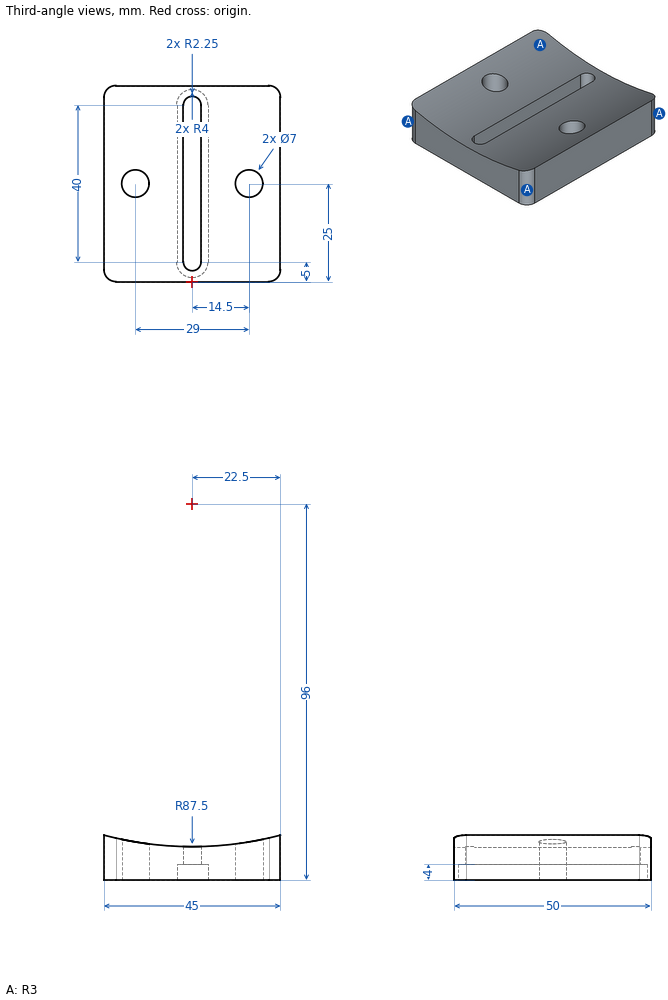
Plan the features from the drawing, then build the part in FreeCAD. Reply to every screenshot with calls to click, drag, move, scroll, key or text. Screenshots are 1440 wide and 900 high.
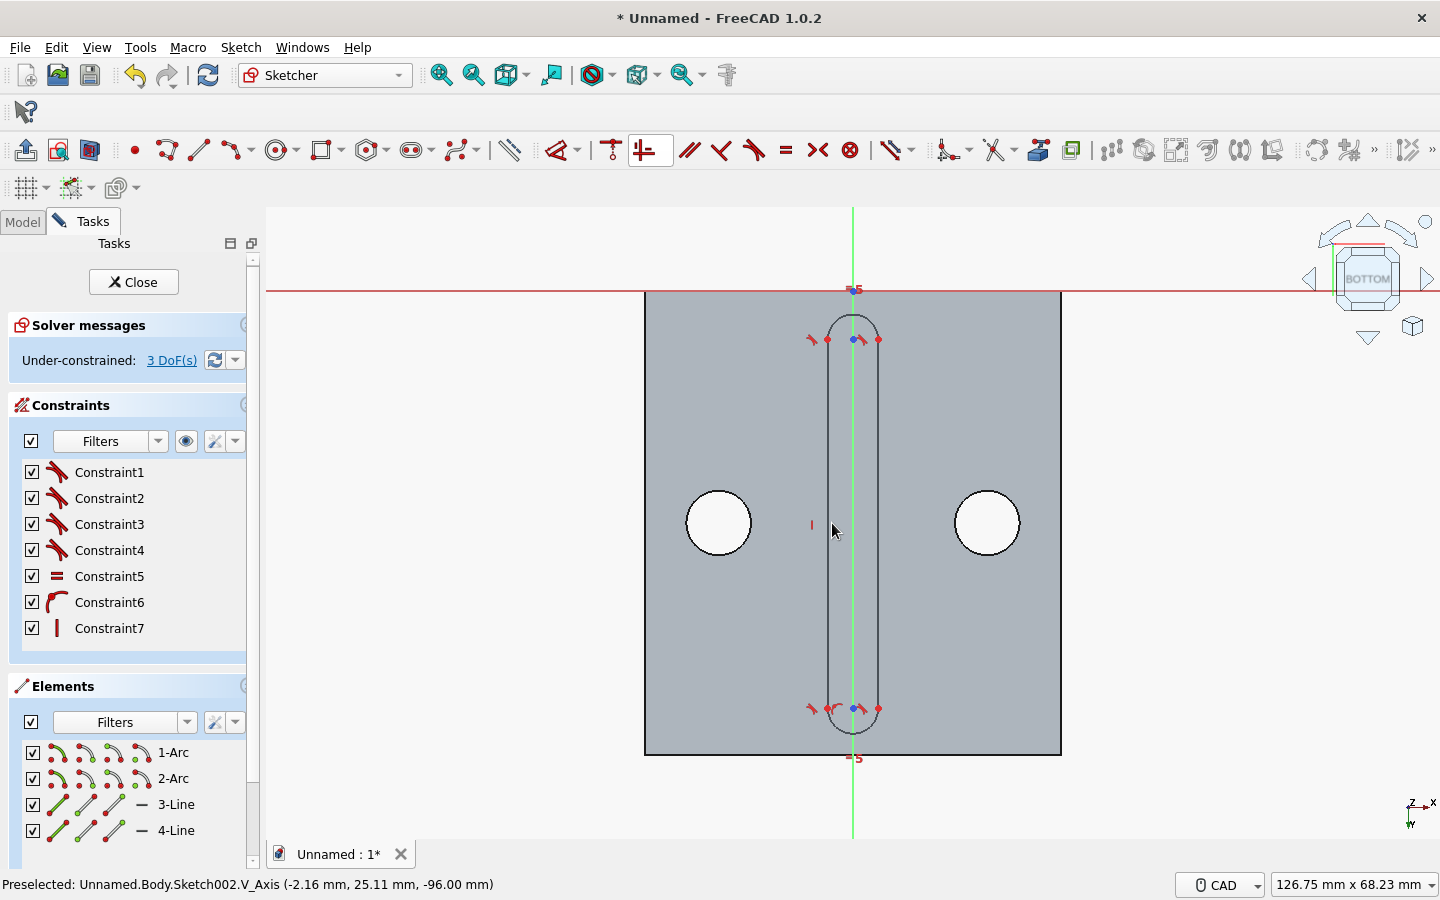
click(556, 150)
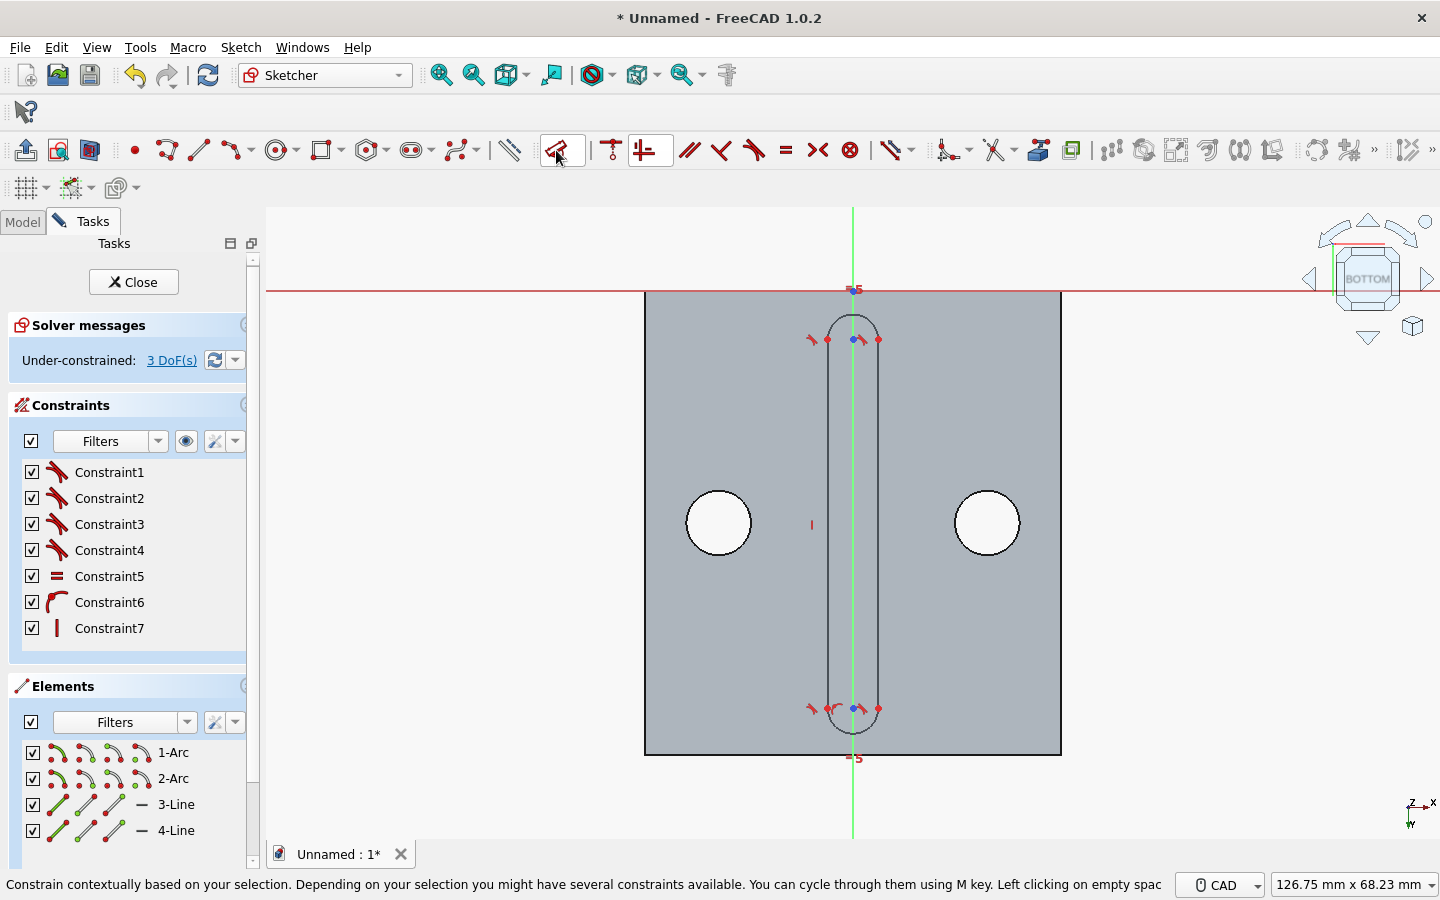
scroll(838, 729, up, 4)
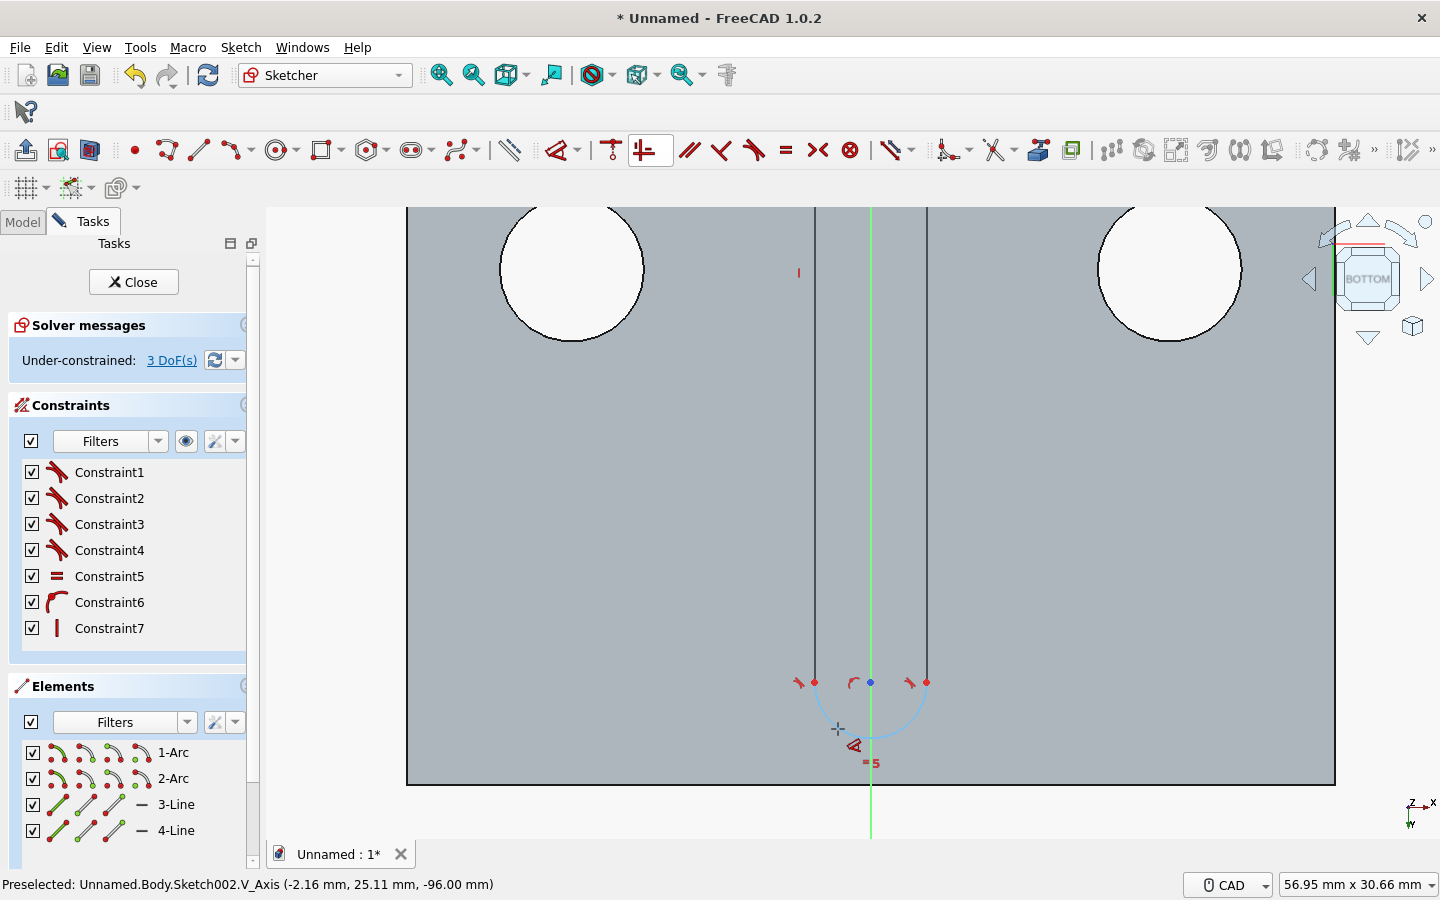
click(838, 728)
click(819, 754)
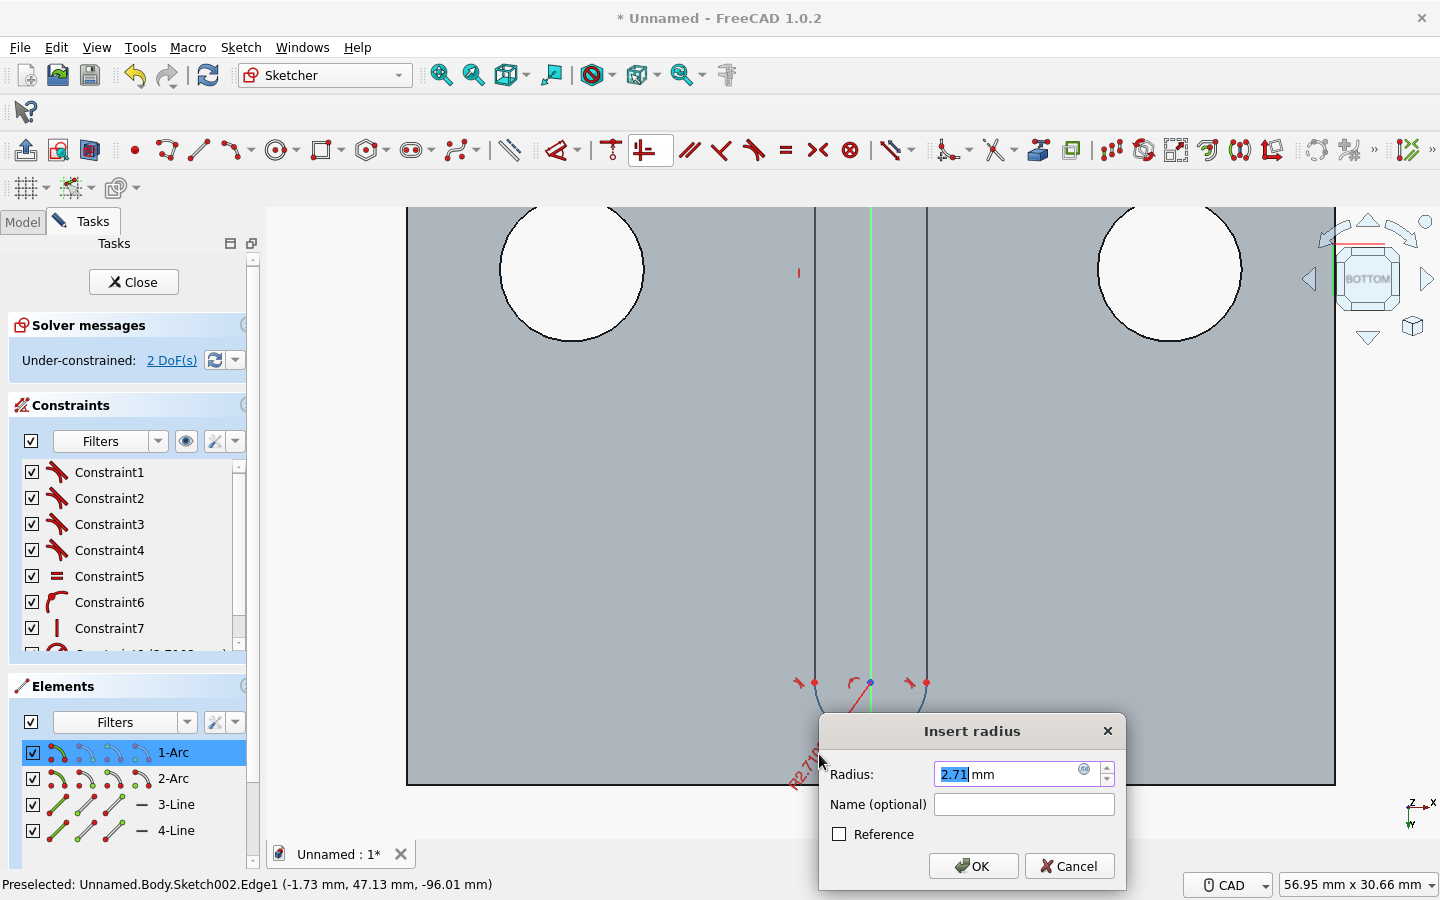
text(2.25)
key(Return)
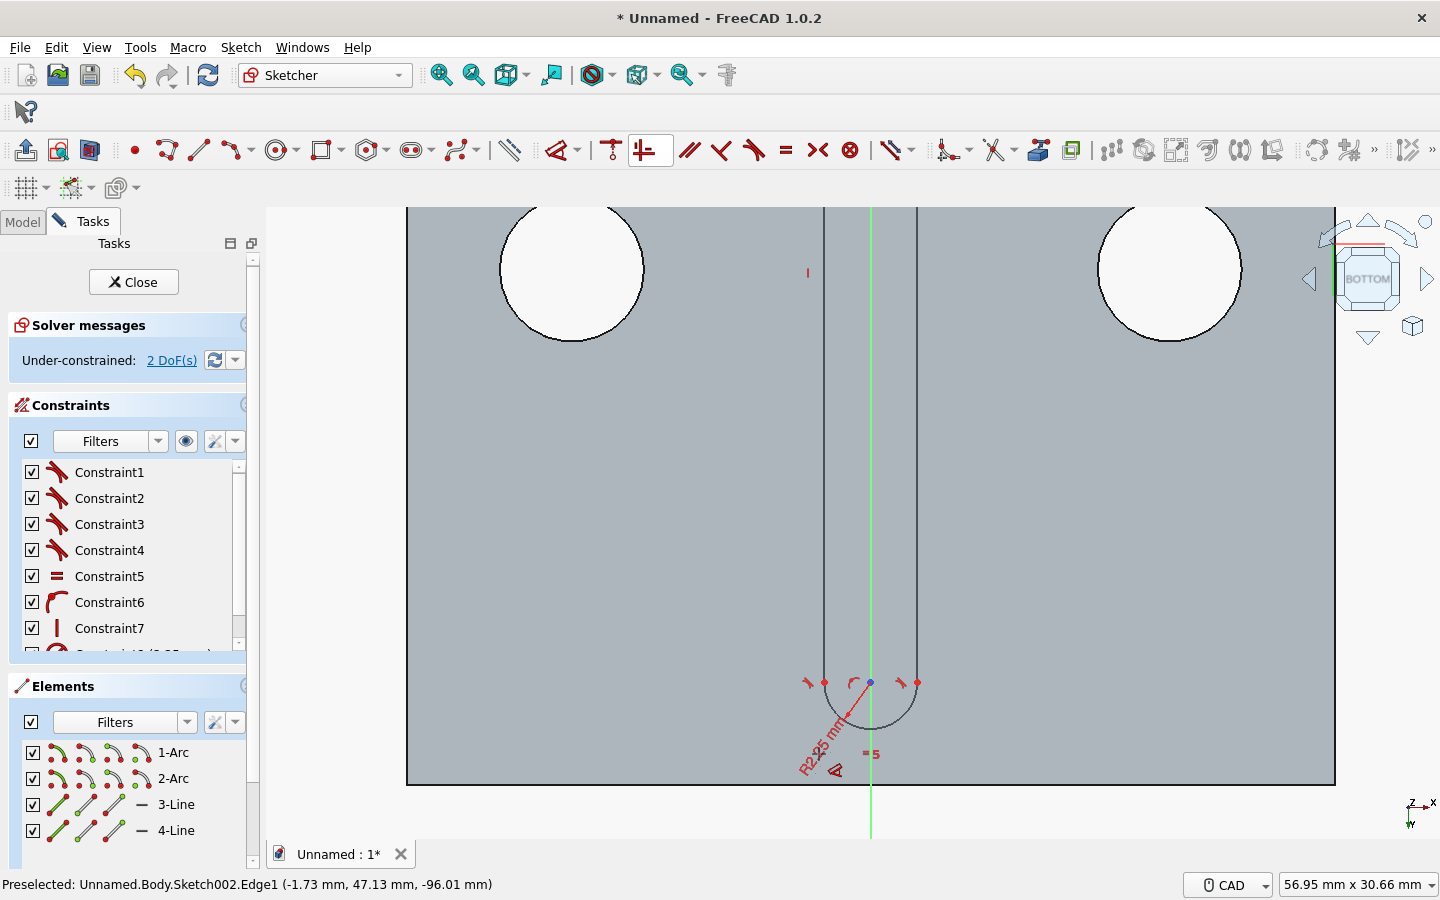
click(824, 436)
click(790, 459)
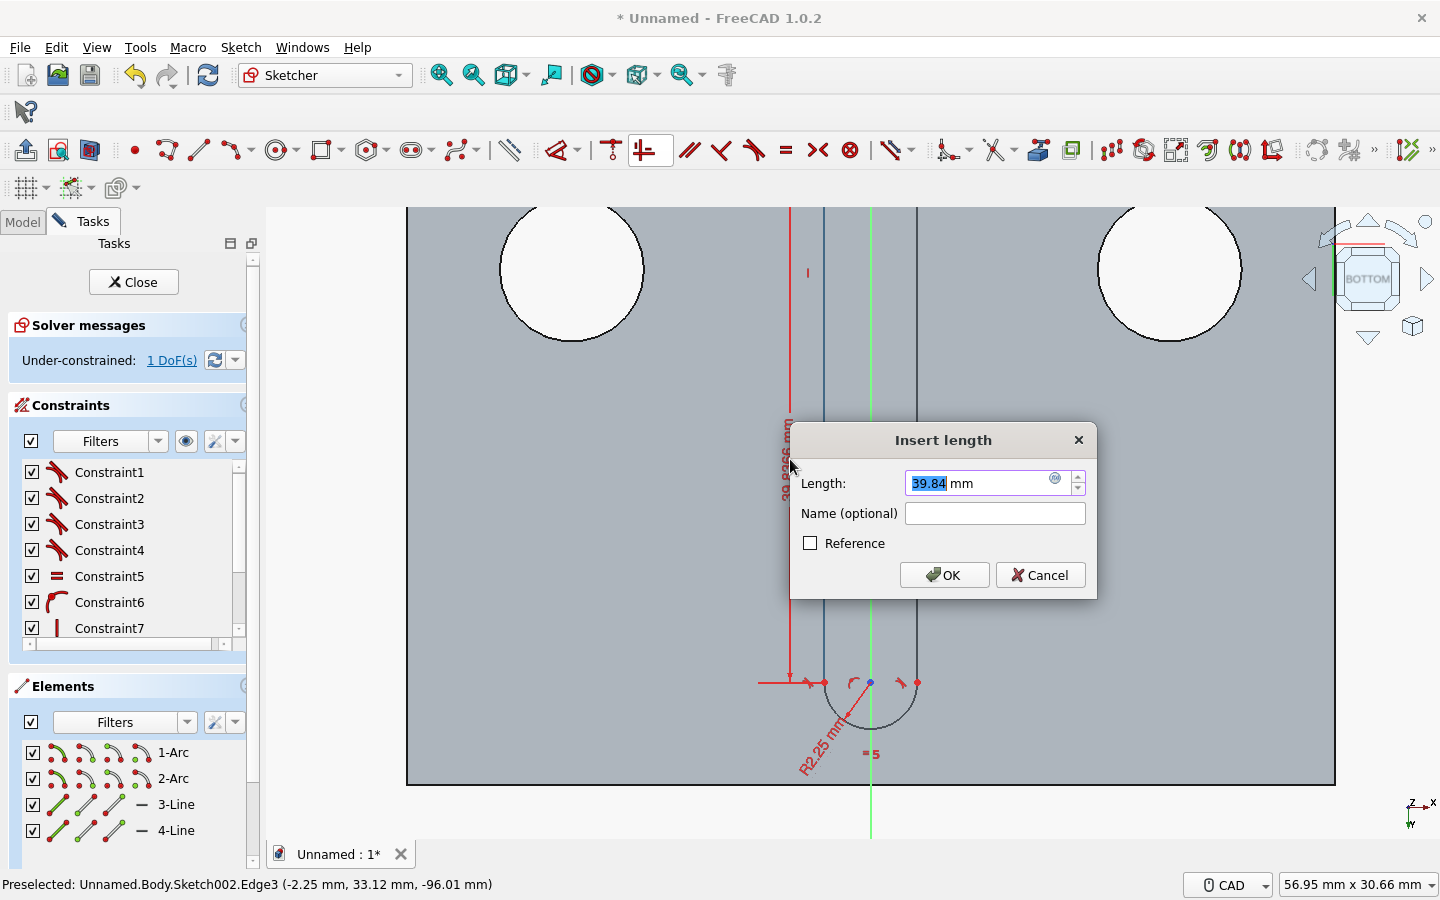
text(40)
key(Return)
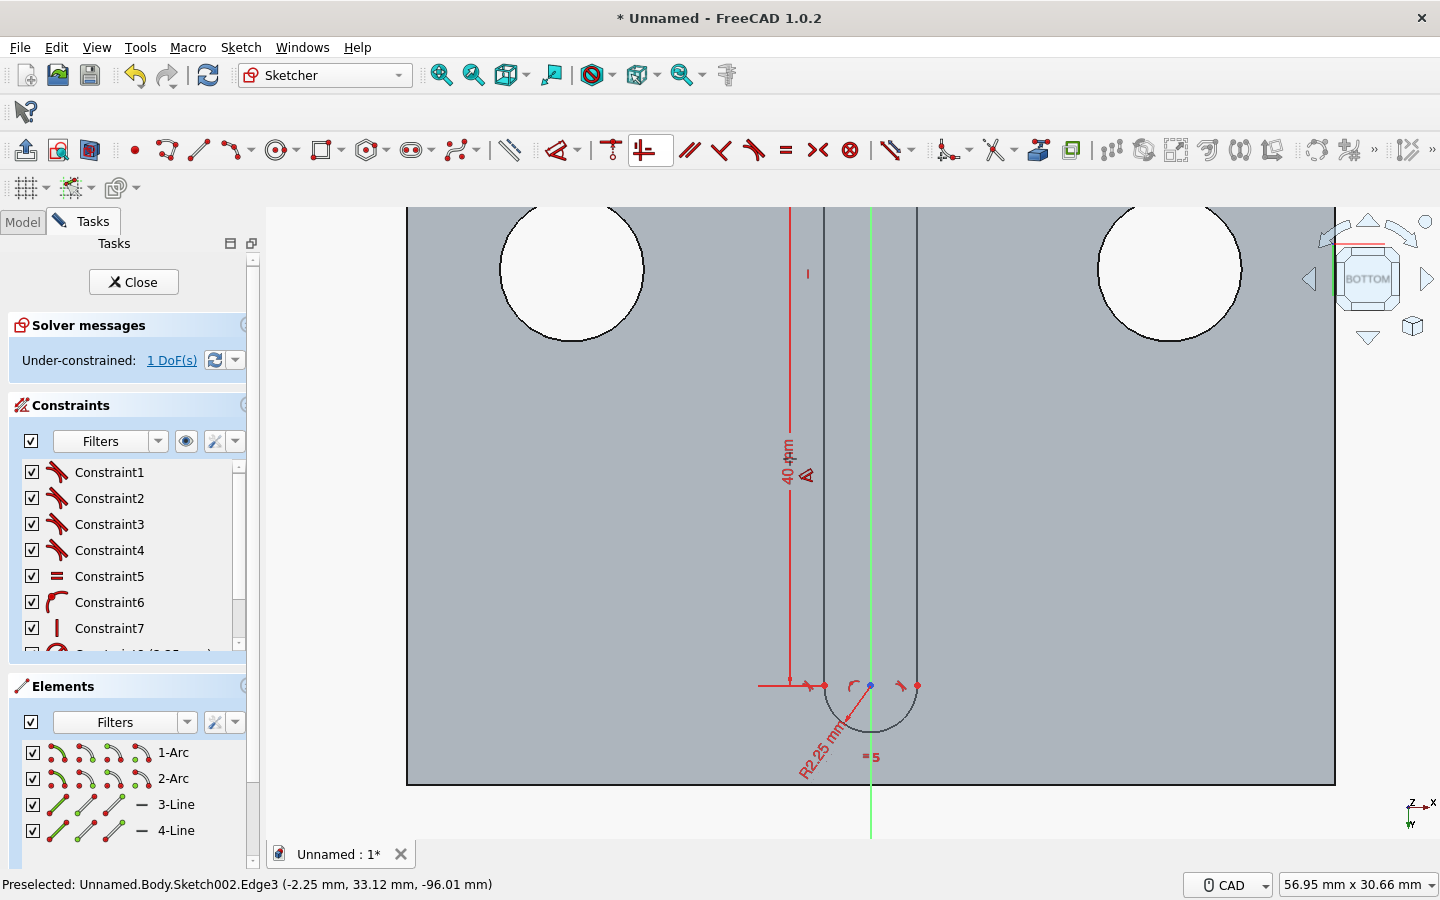
scroll(714, 753, down, 4)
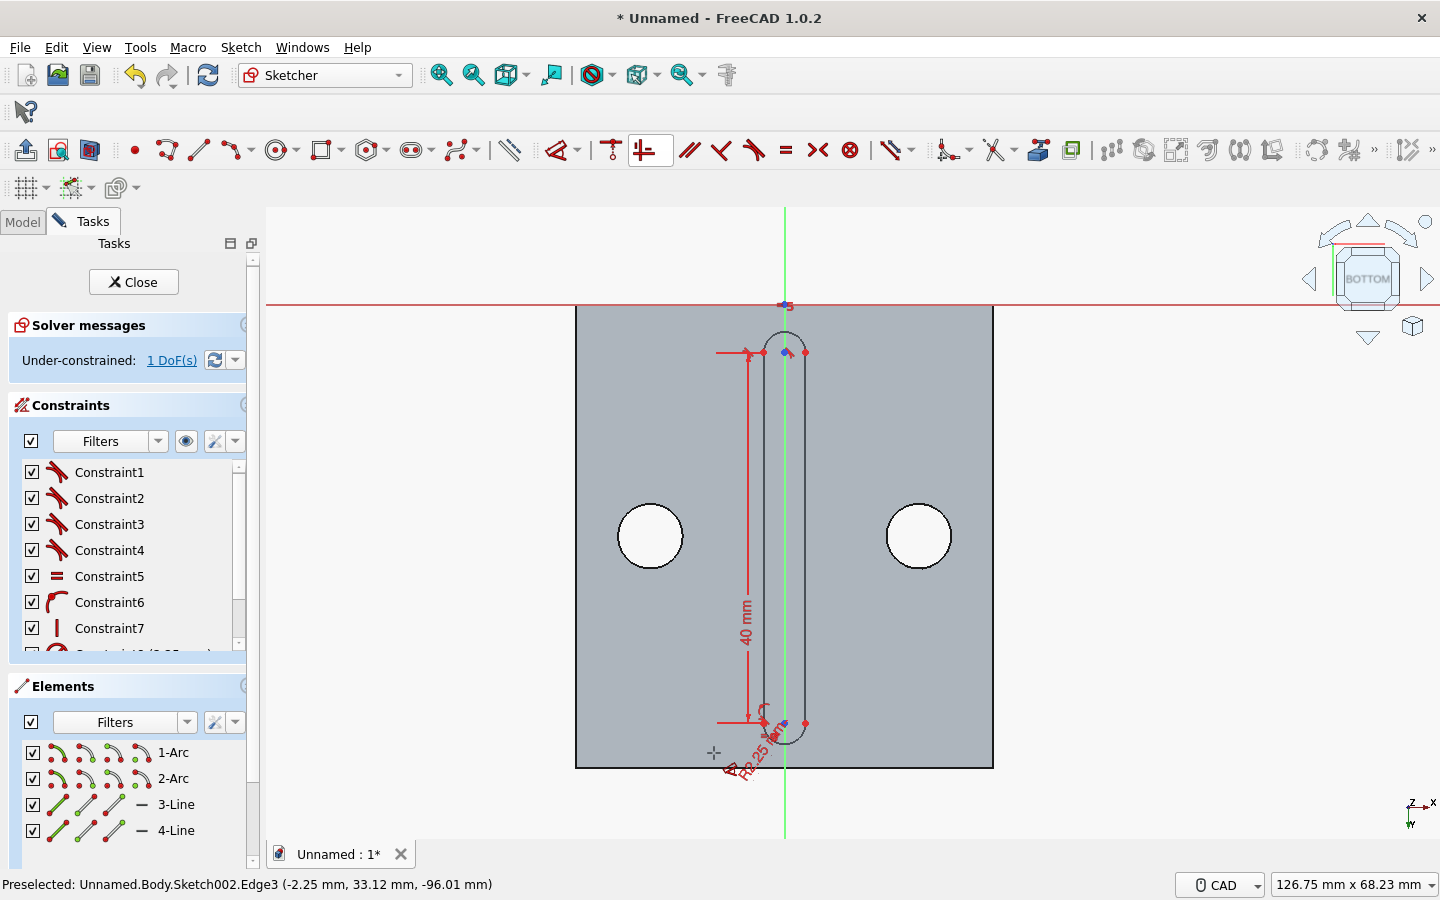
click(805, 353)
click(839, 329)